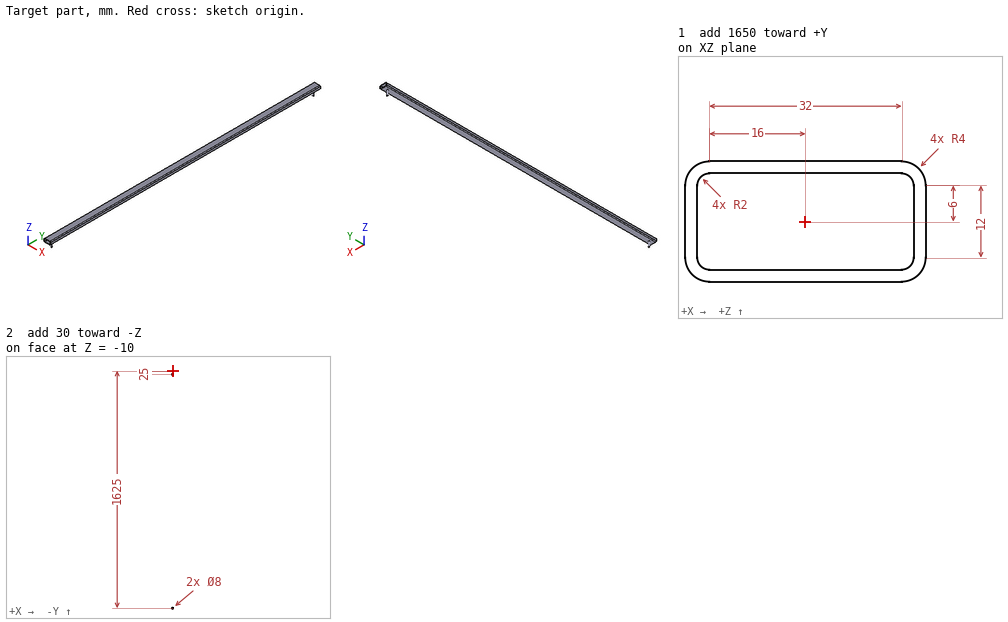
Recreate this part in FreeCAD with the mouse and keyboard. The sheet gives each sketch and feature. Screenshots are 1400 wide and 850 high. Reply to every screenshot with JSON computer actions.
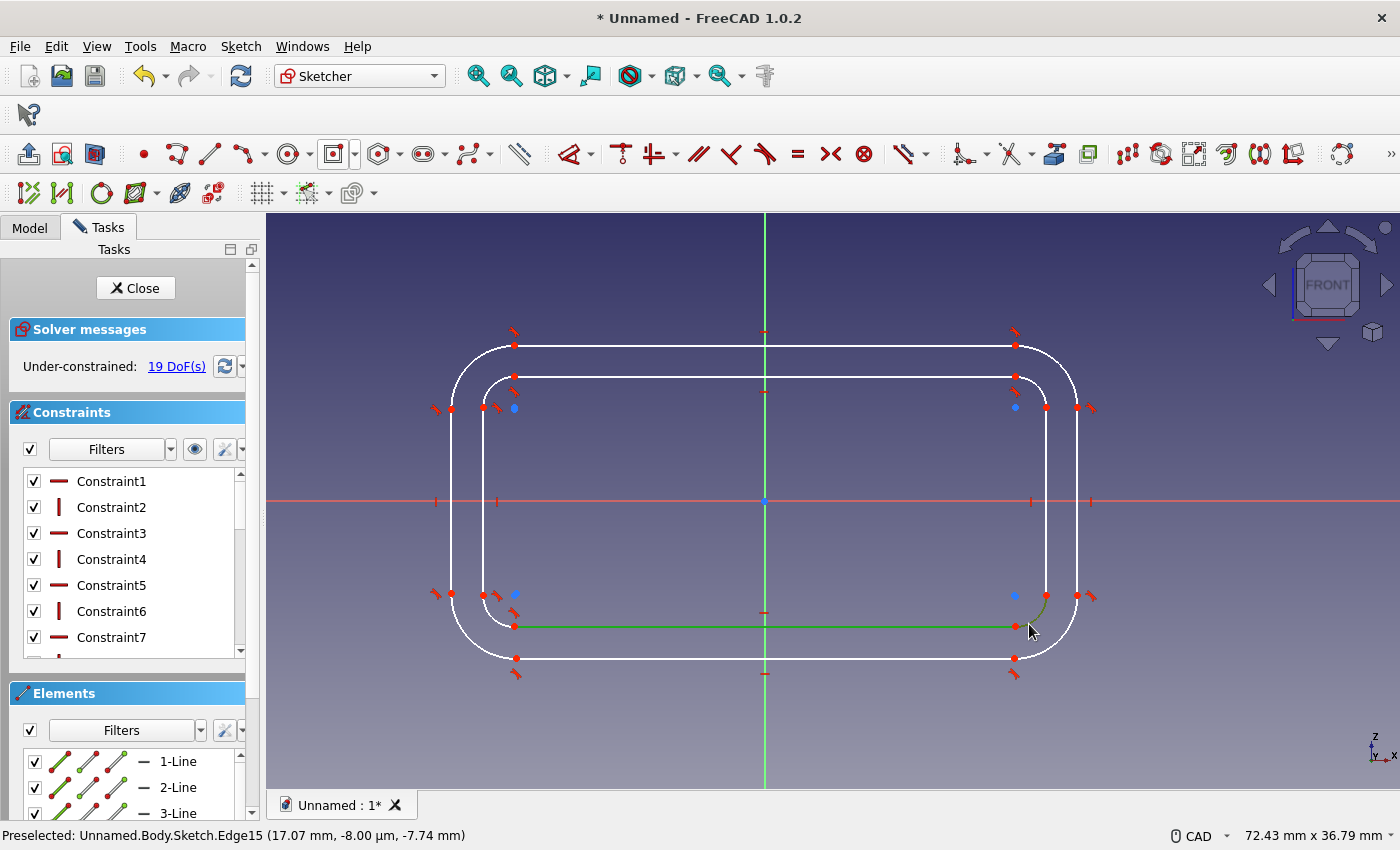
{"action": "left_click", "coordinate": [765, 154]}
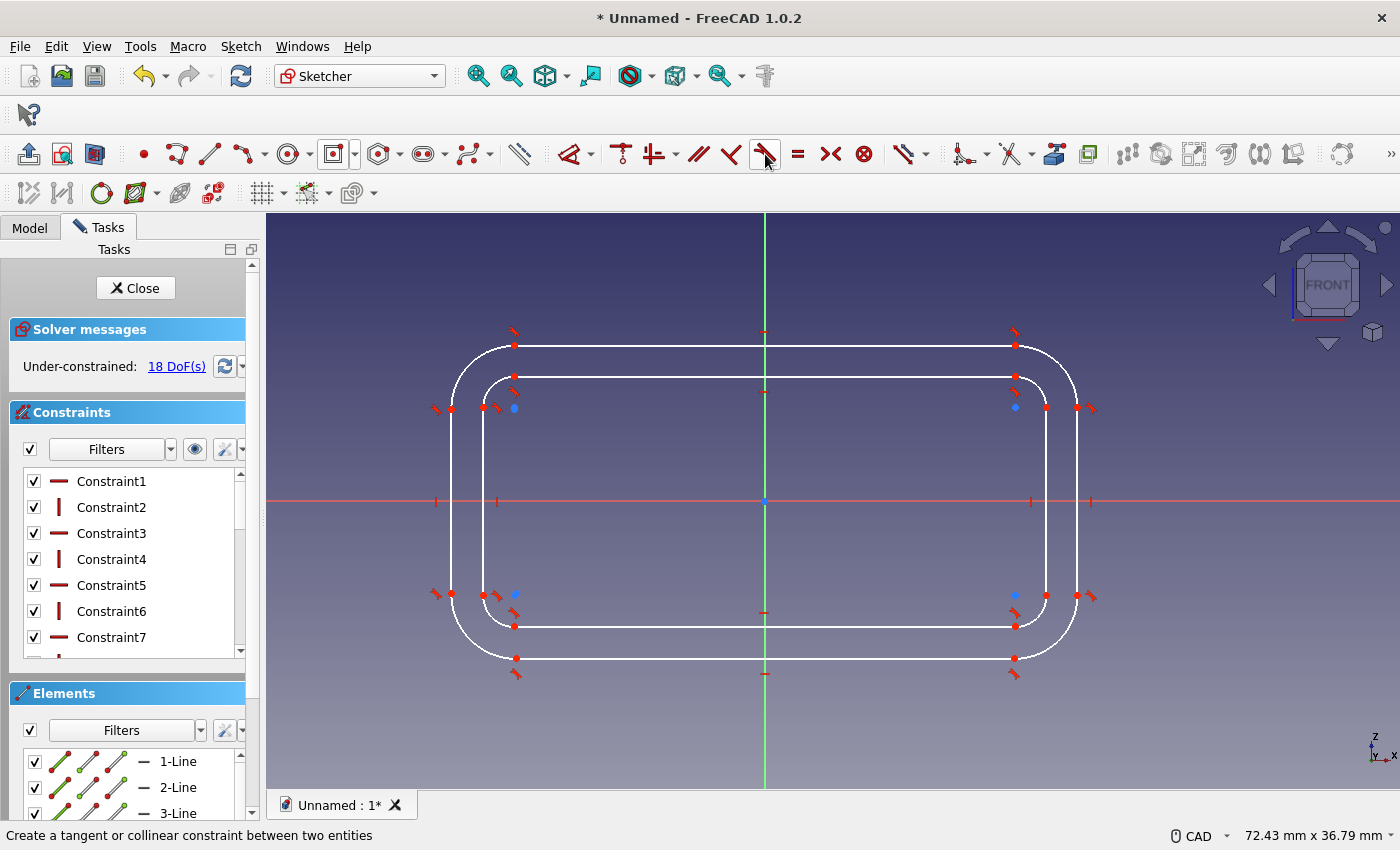
{"action": "left_click", "coordinate": [1046, 540]}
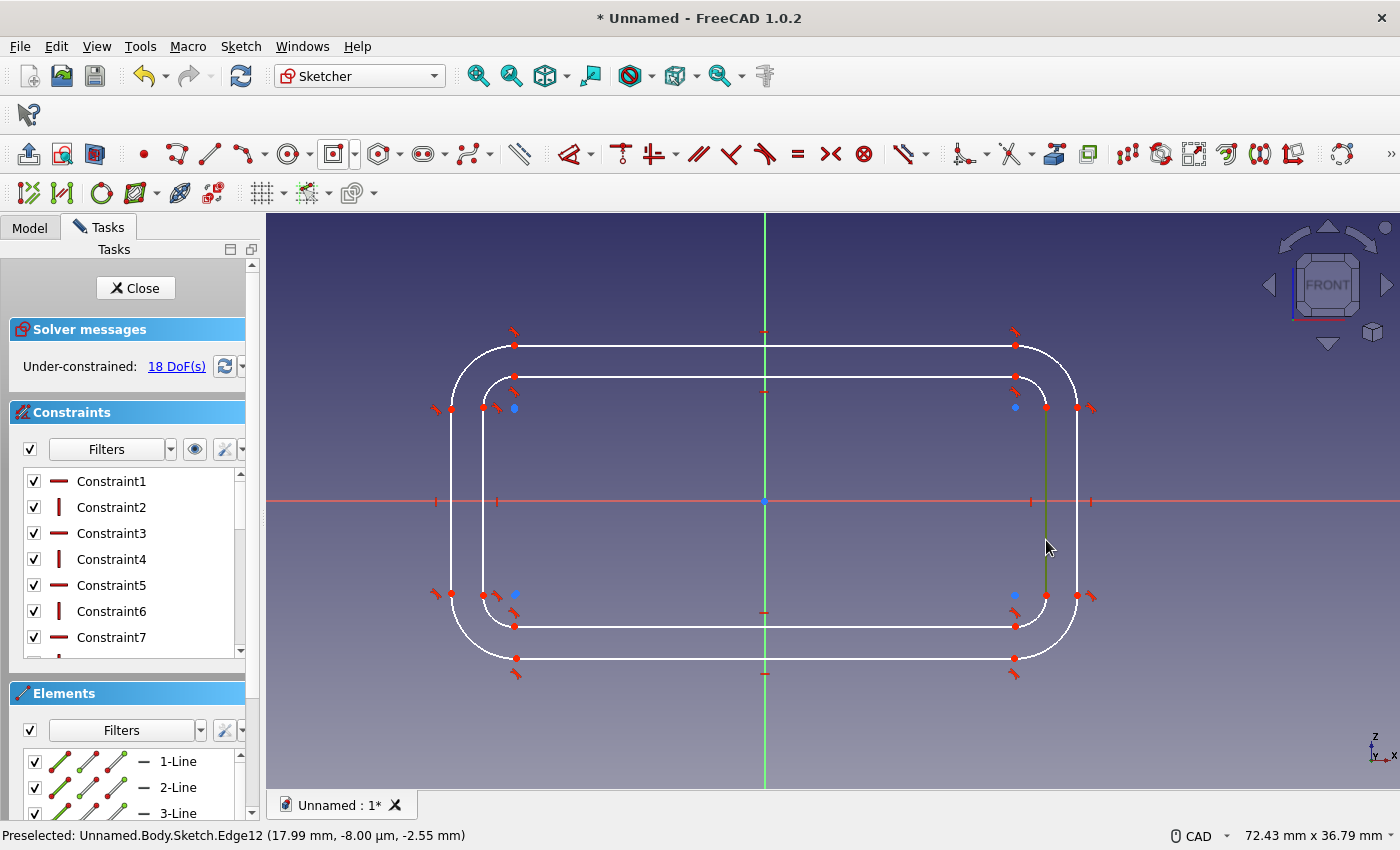
{"action": "left_click", "coordinate": [1029, 624]}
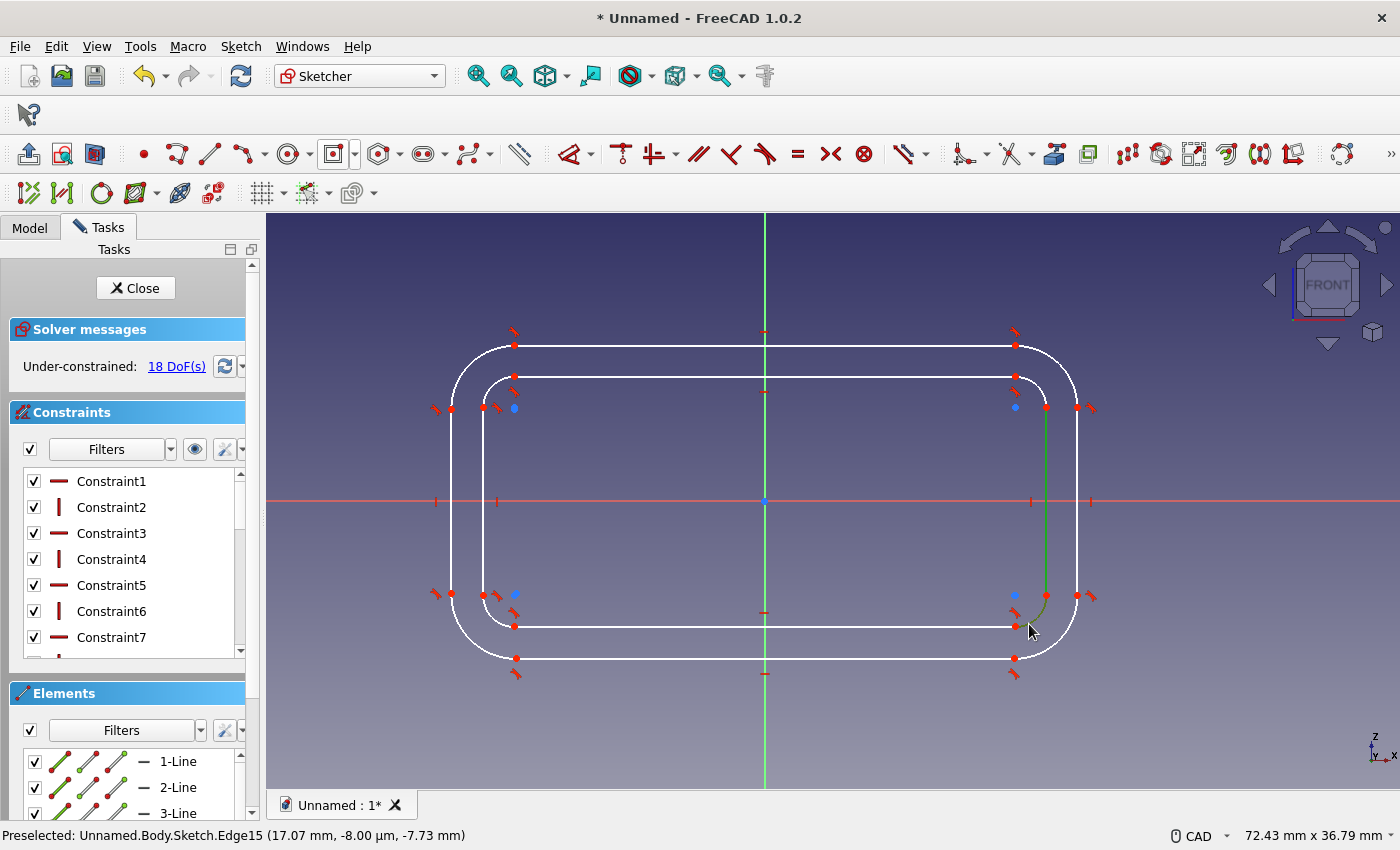
{"action": "left_click", "coordinate": [765, 154]}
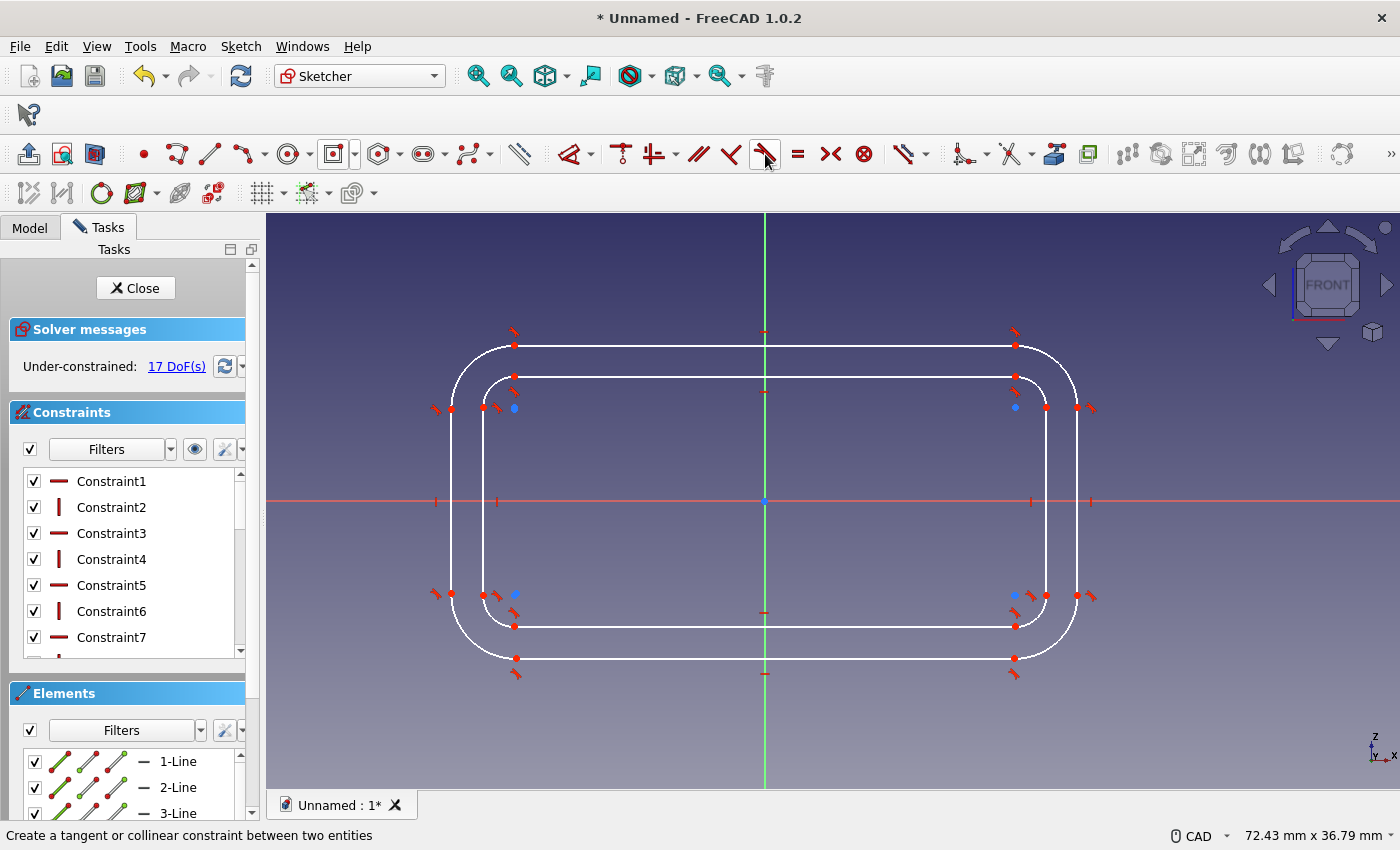
{"action": "left_click", "coordinate": [1046, 540]}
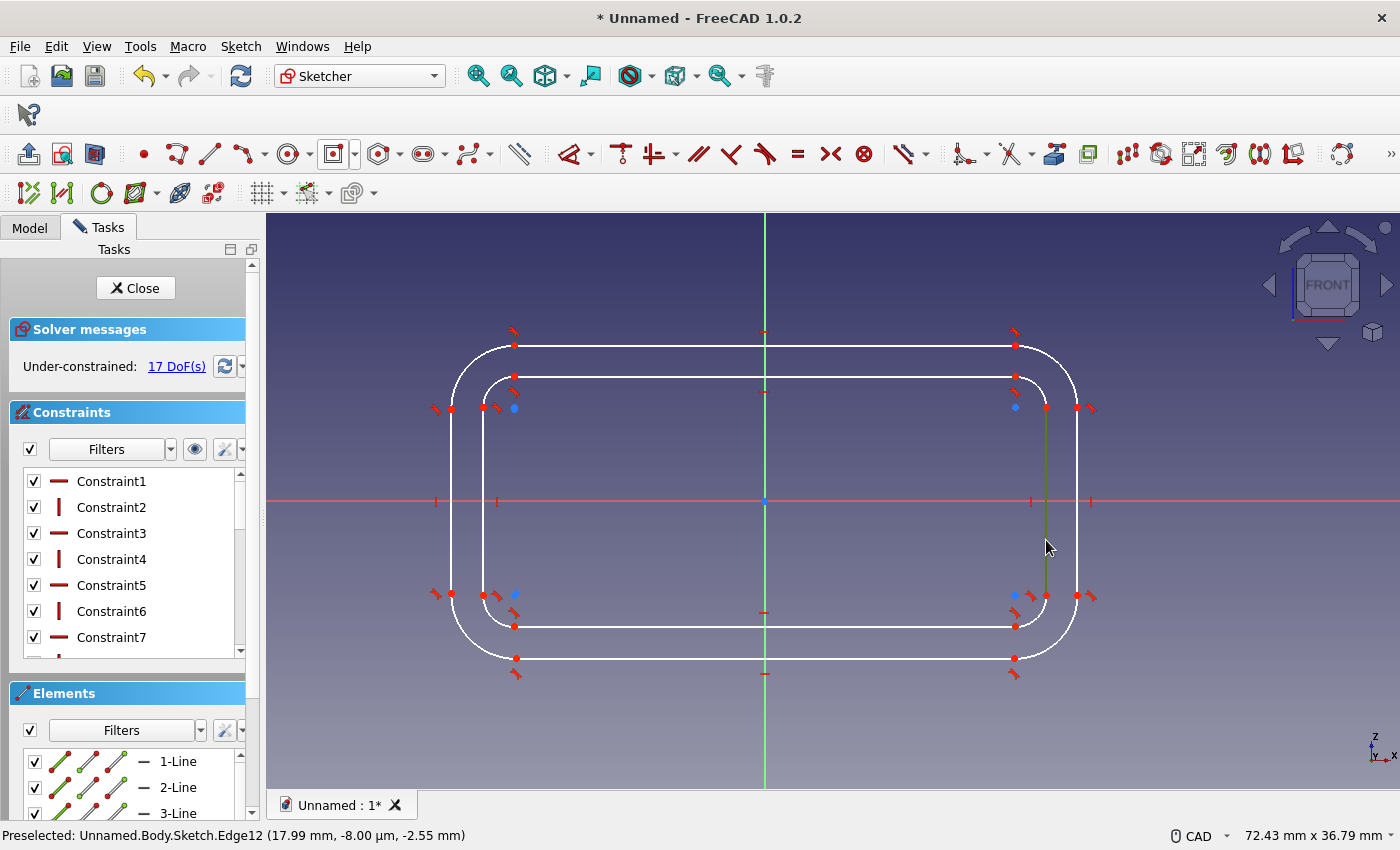
{"action": "left_click", "coordinate": [1043, 394]}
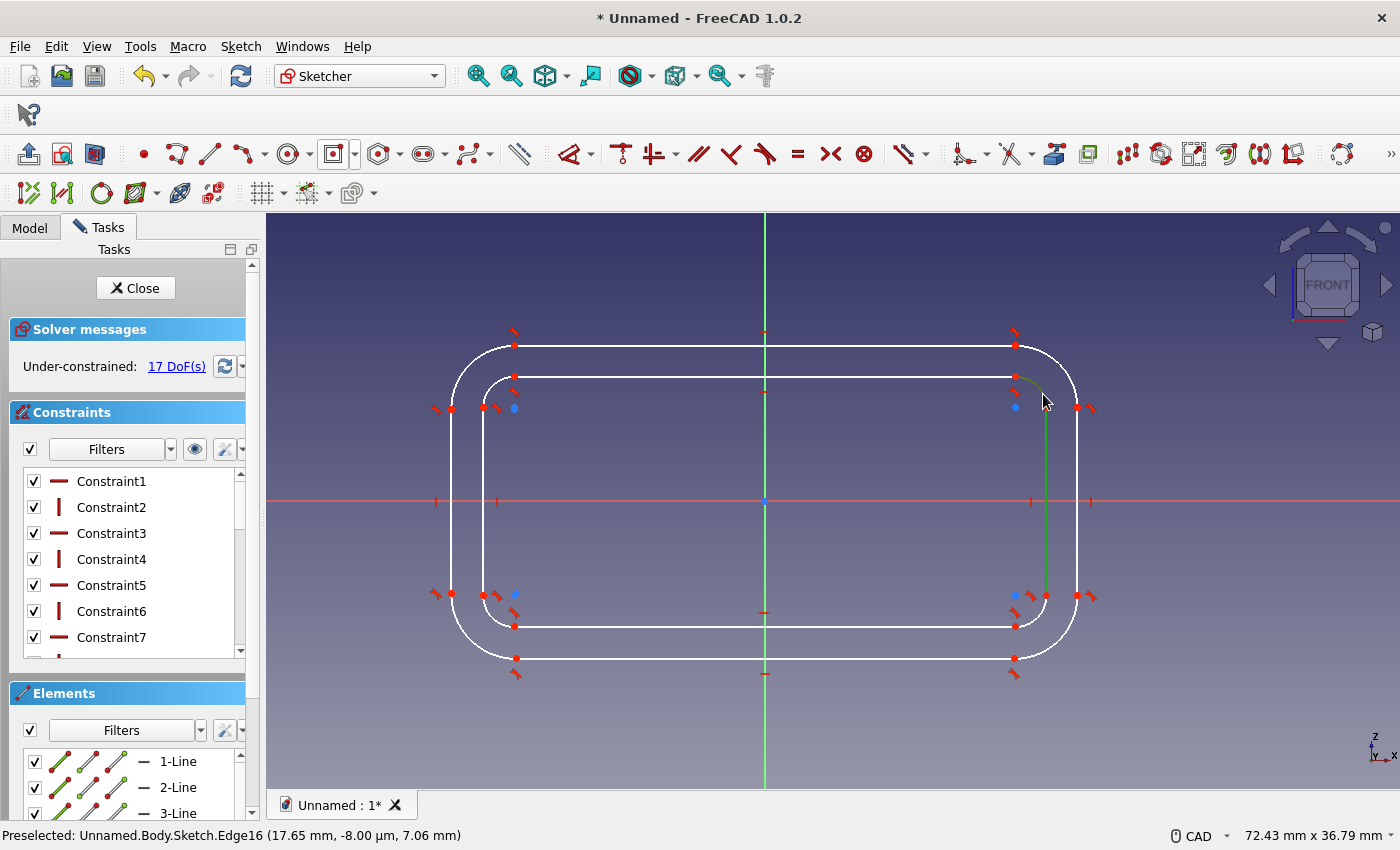
{"action": "left_click", "coordinate": [765, 154]}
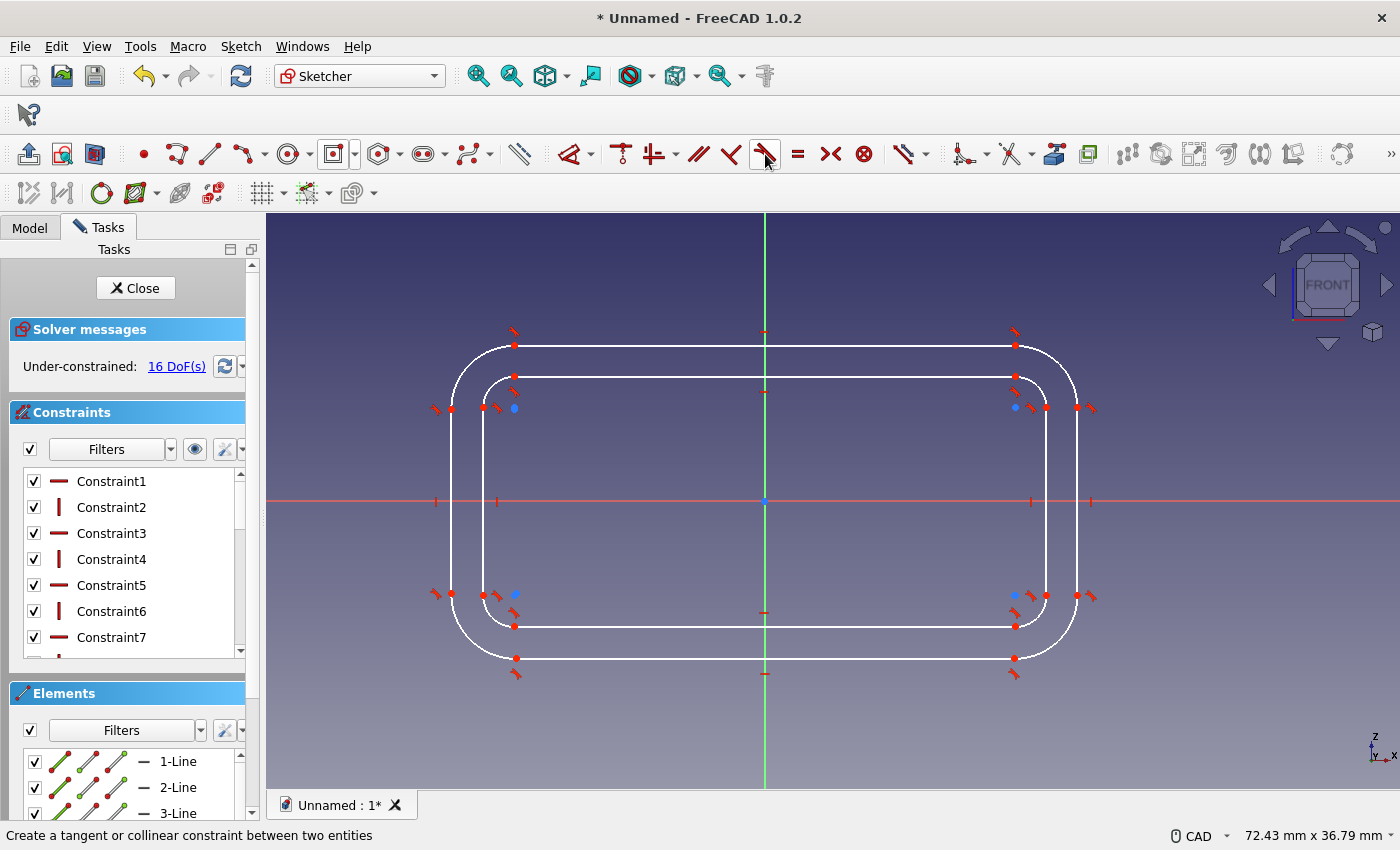
{"action": "left_click", "coordinate": [486, 353]}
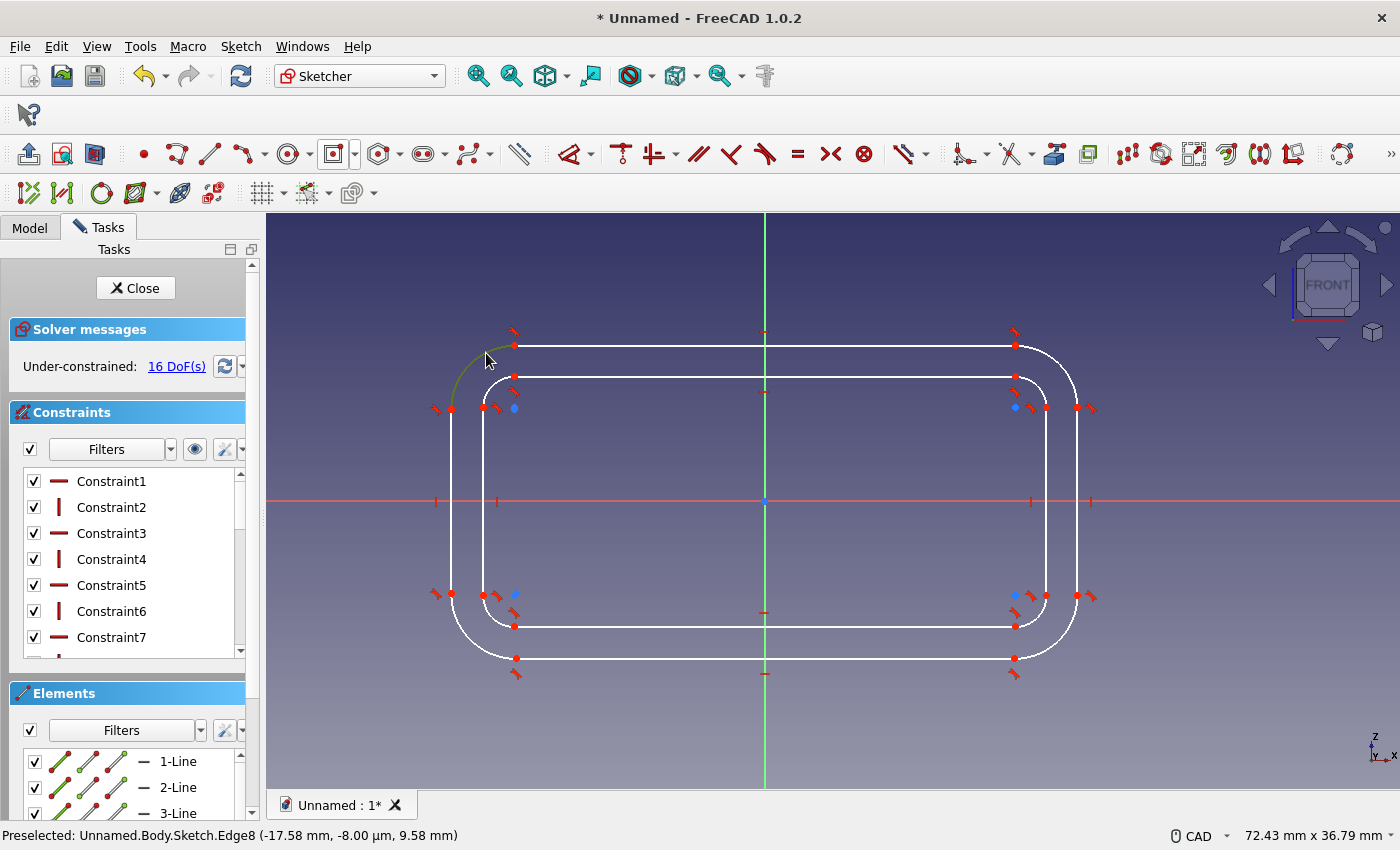
{"action": "left_click", "coordinate": [500, 380]}